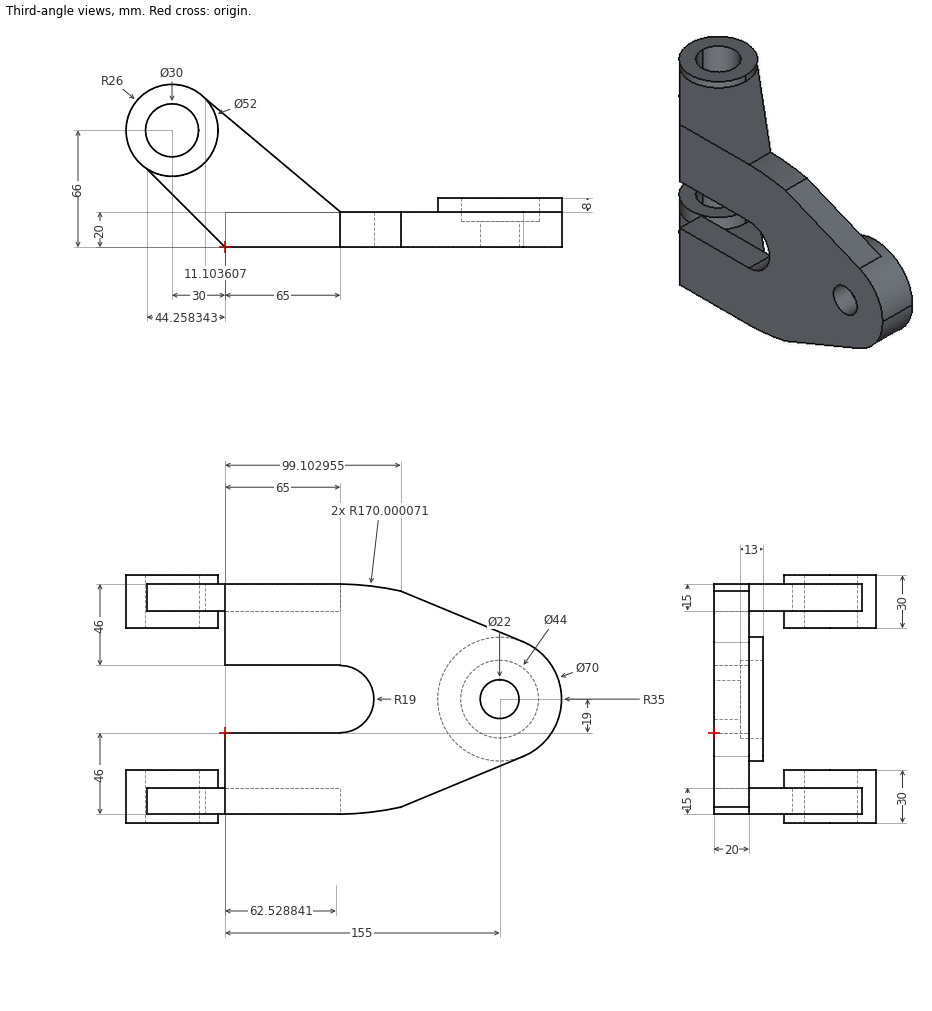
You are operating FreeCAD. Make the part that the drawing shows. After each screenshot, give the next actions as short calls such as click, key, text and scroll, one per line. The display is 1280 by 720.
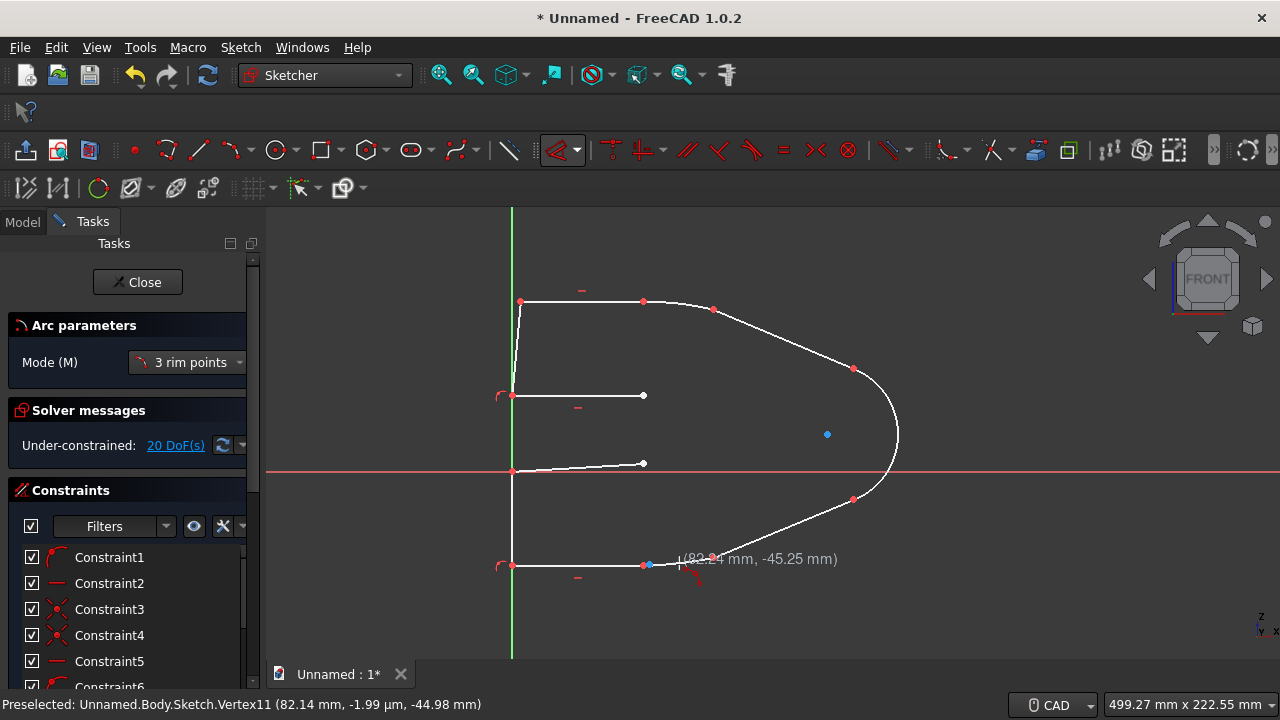
click(644, 464)
click(644, 396)
click(683, 433)
key(Escape)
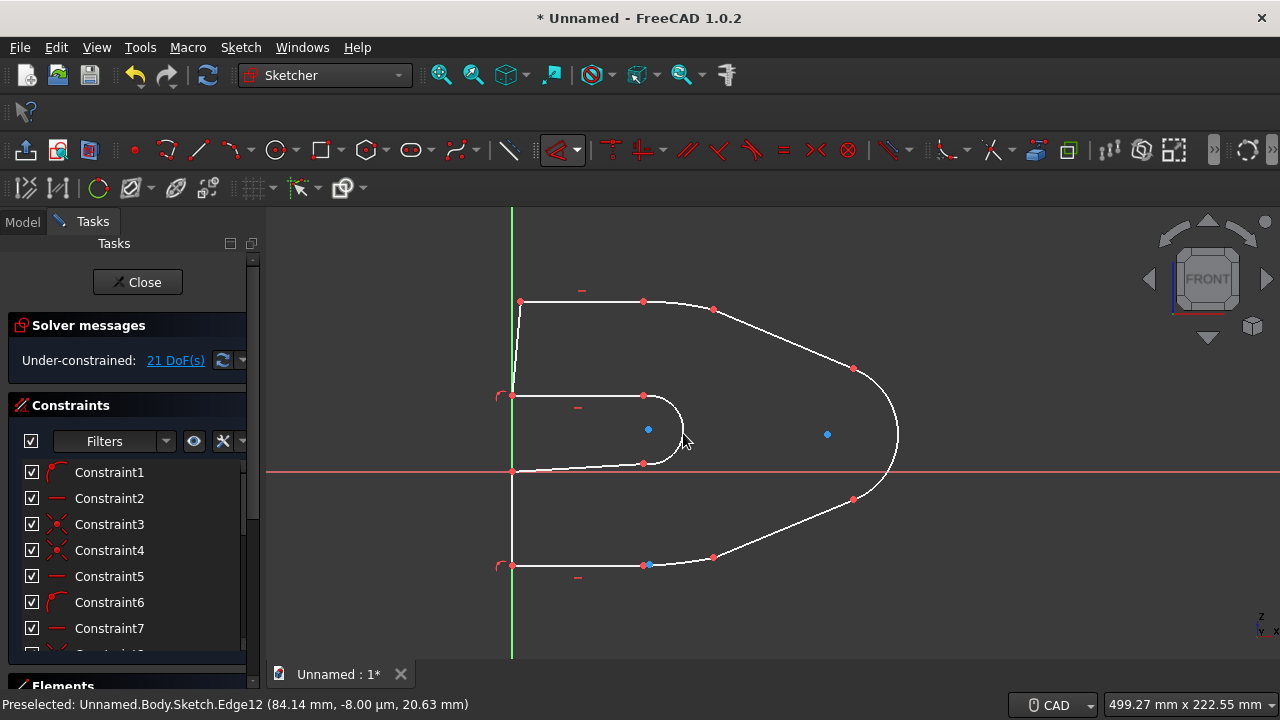
click(604, 396)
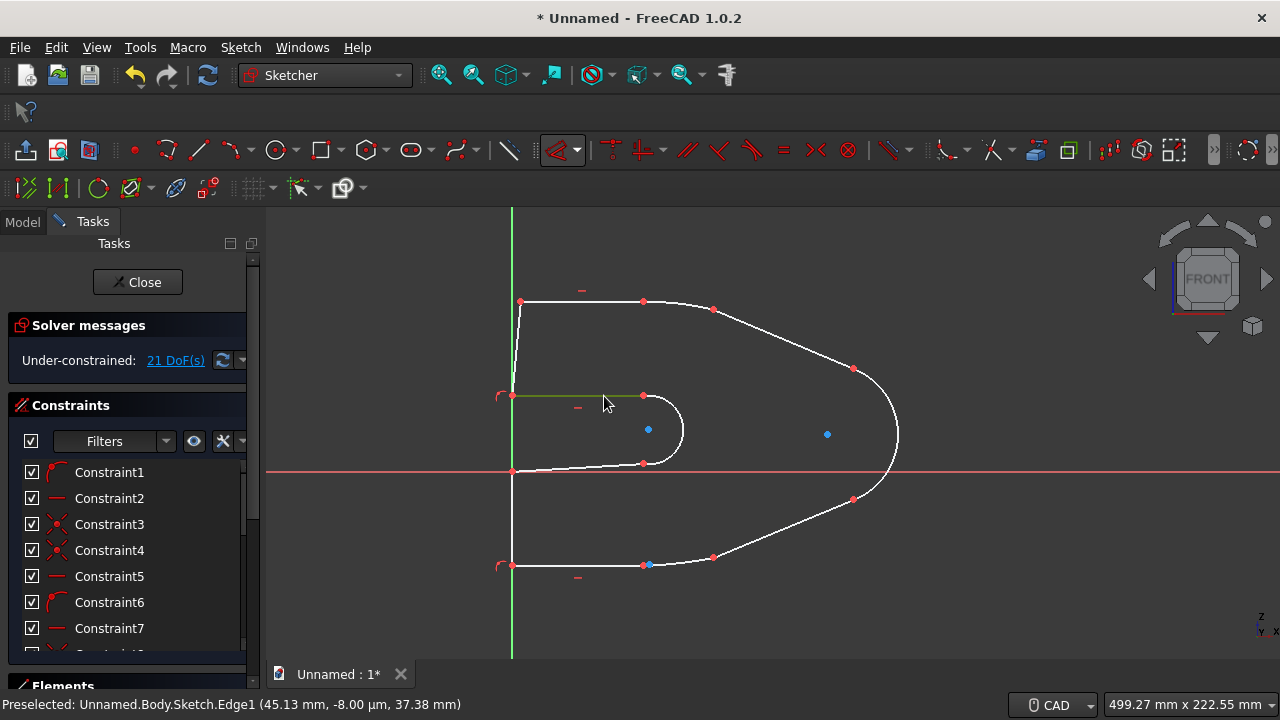
click(675, 452)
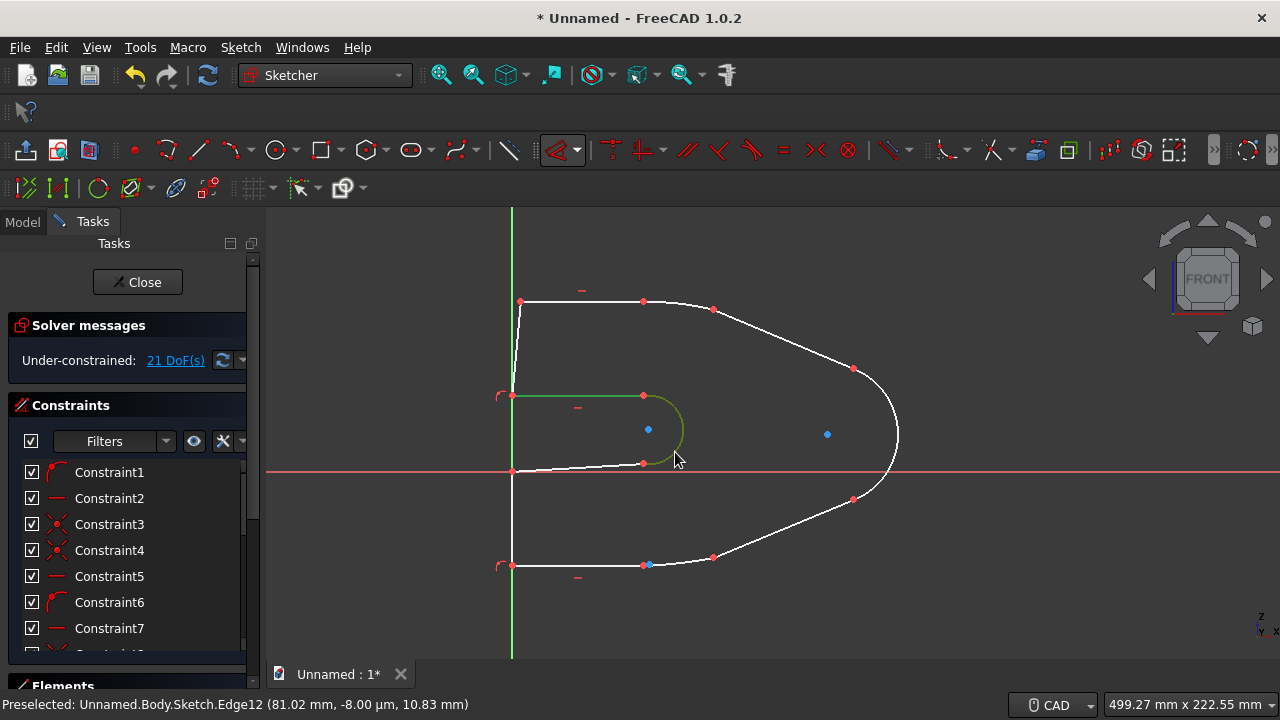
key(t)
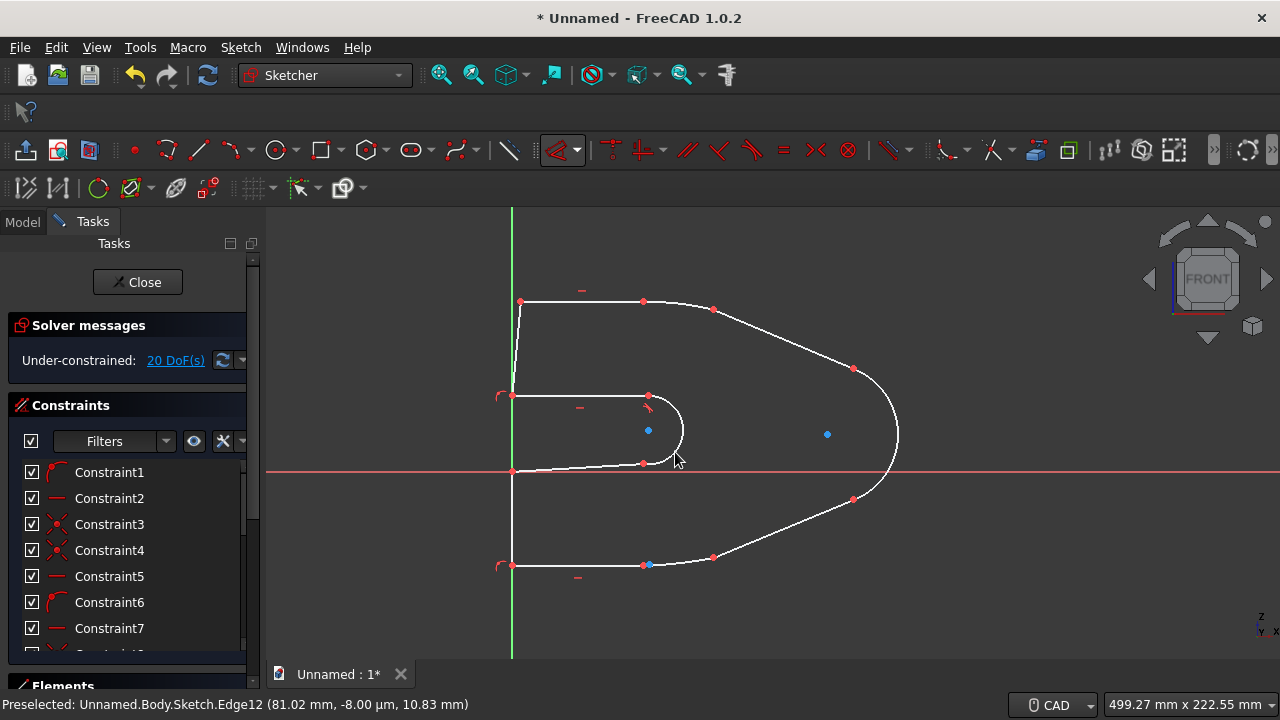
click(756, 328)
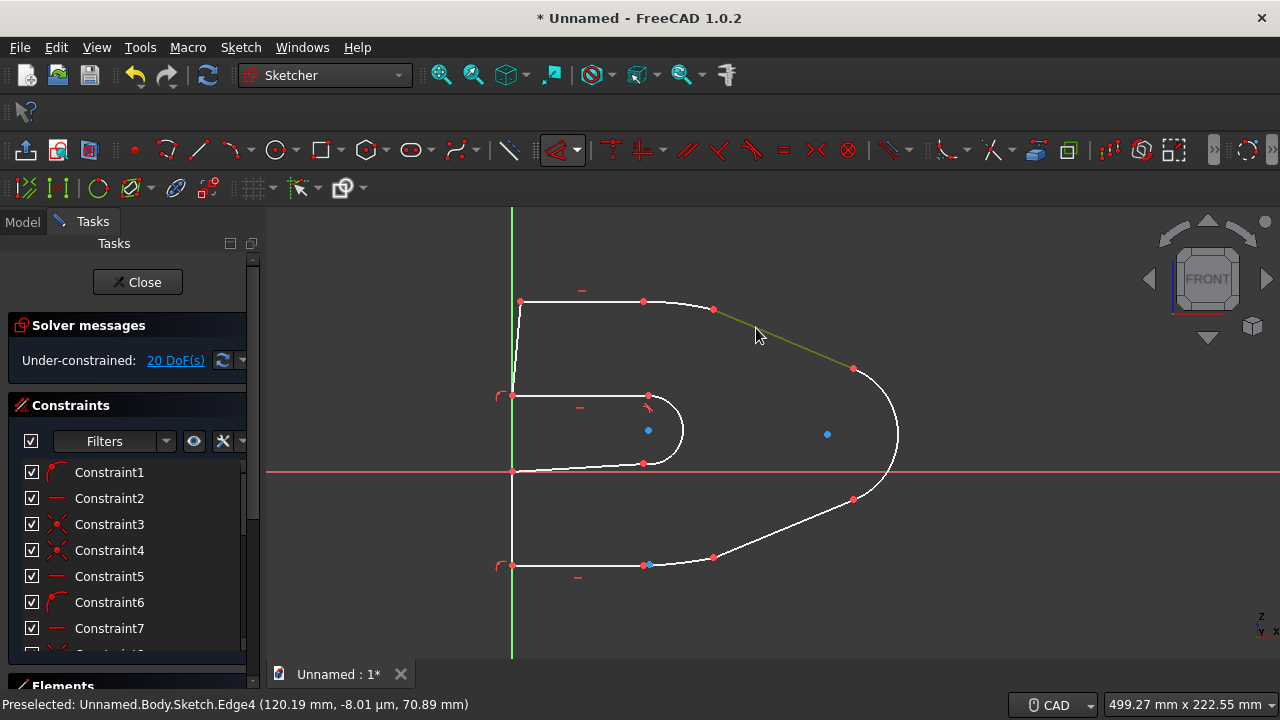
click(890, 402)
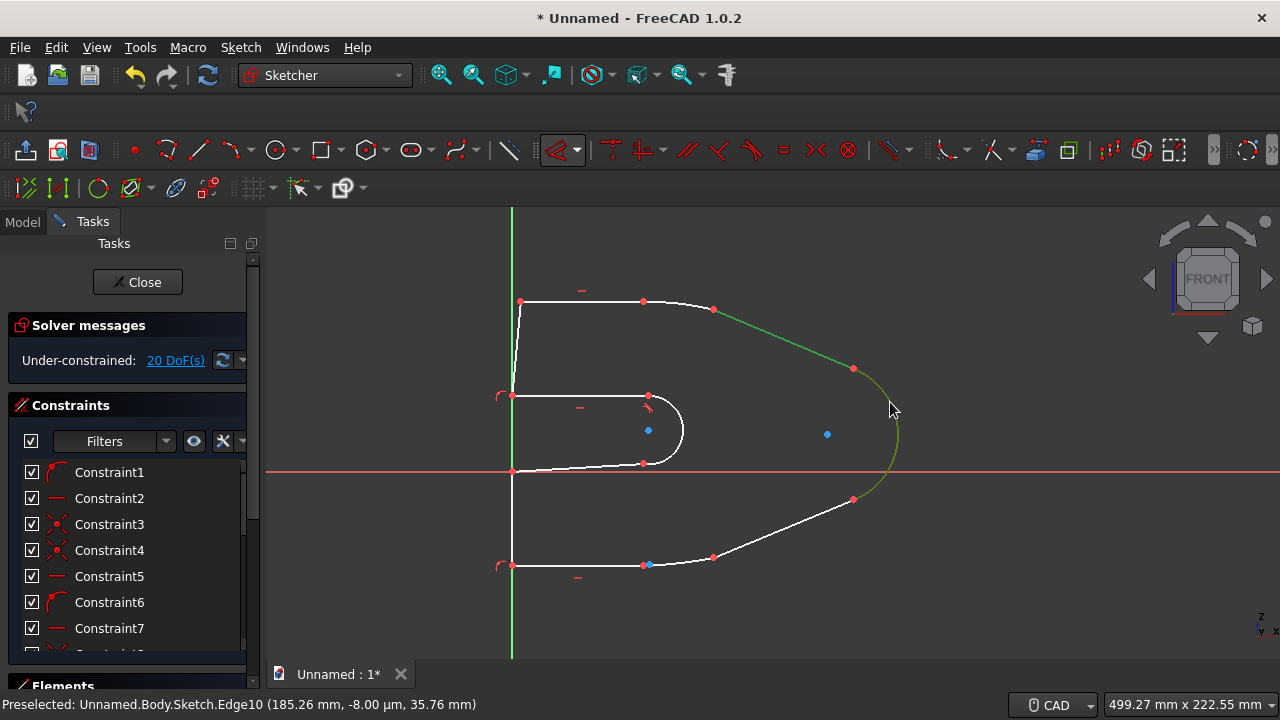
click(752, 150)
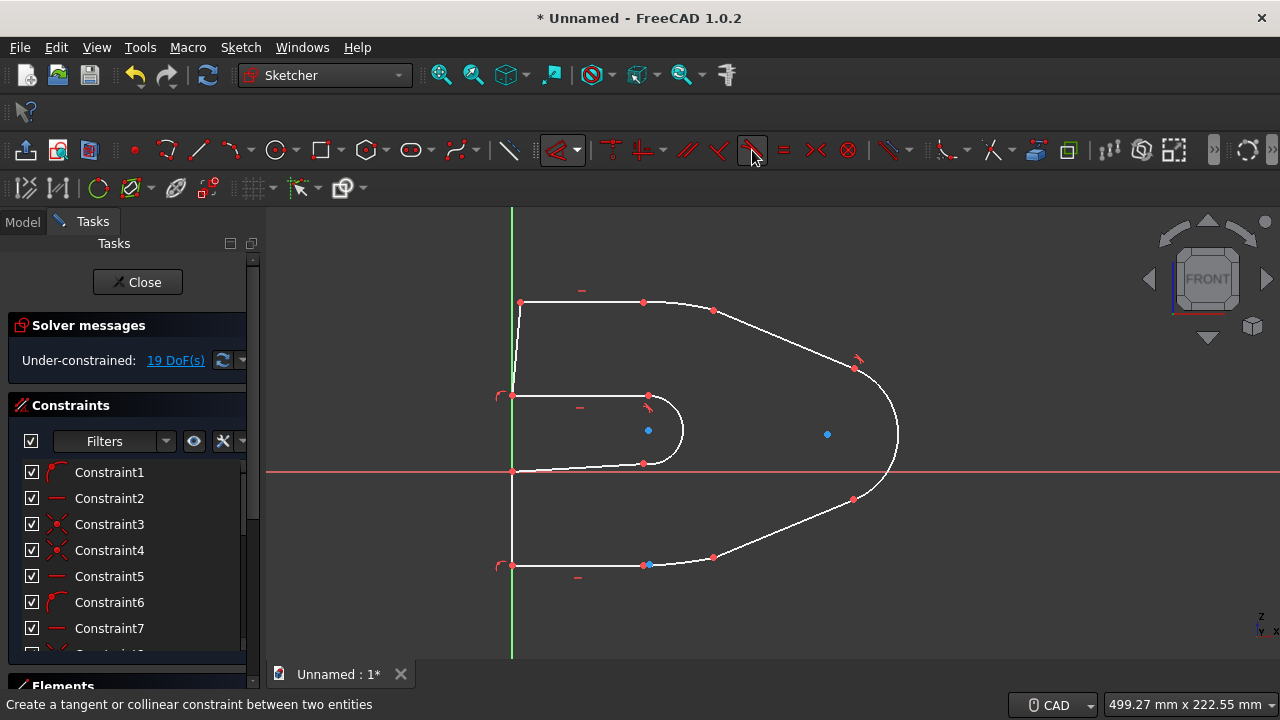
click(812, 517)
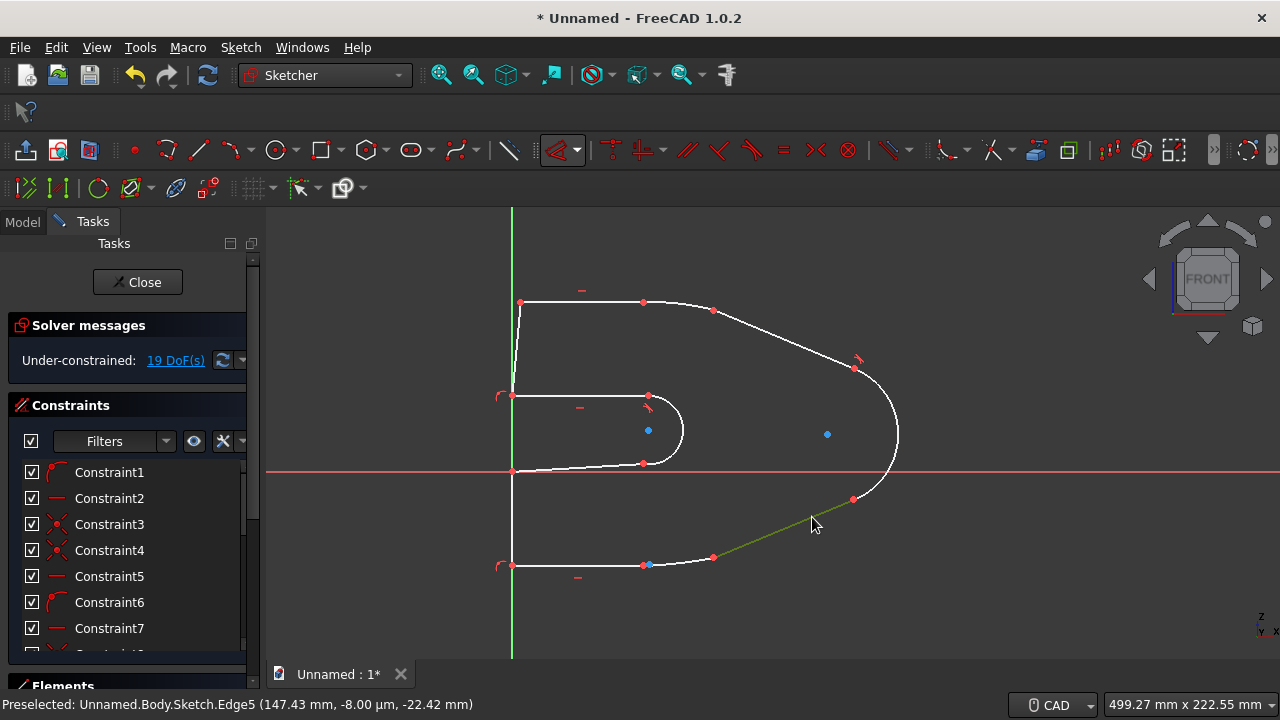
click(891, 403)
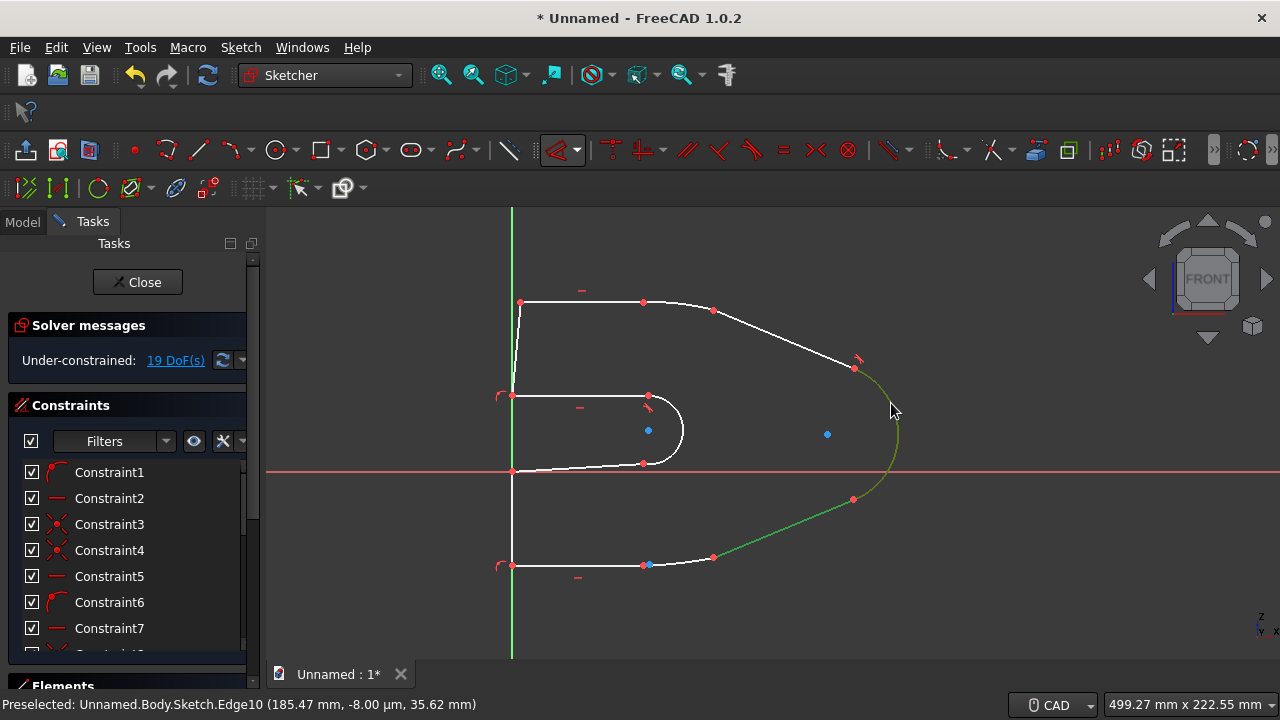
click(752, 150)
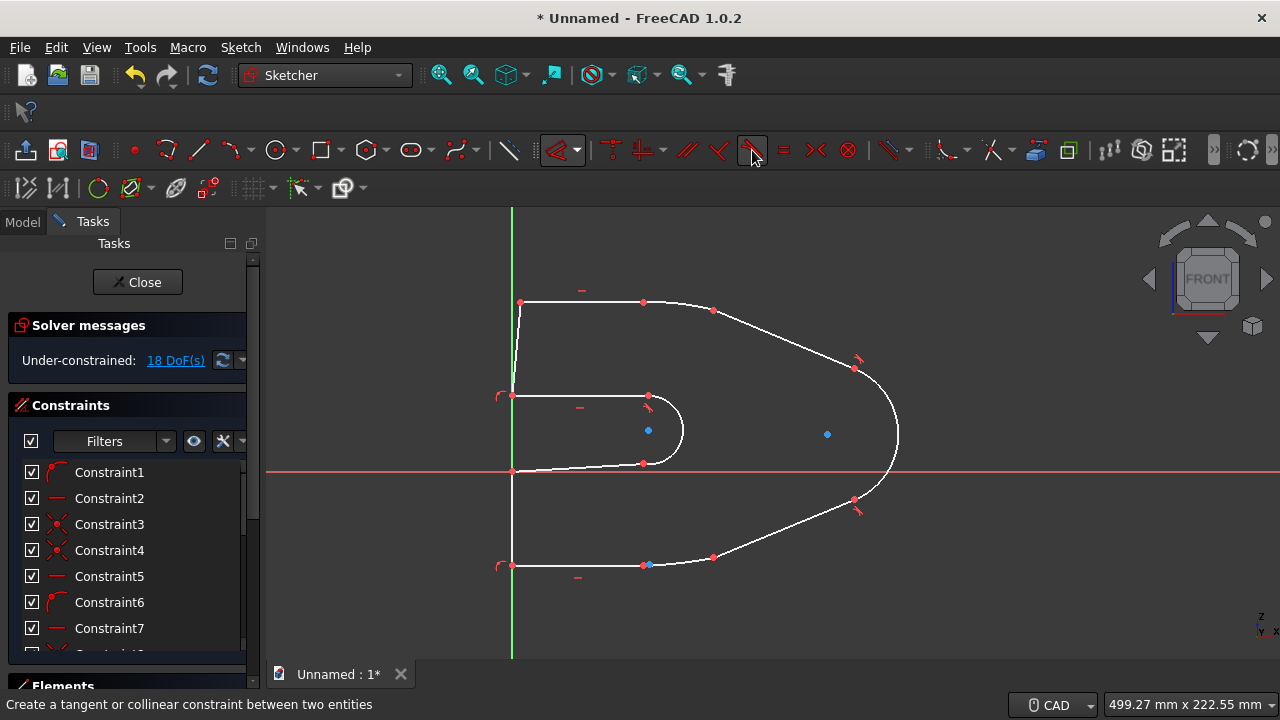
click(552, 470)